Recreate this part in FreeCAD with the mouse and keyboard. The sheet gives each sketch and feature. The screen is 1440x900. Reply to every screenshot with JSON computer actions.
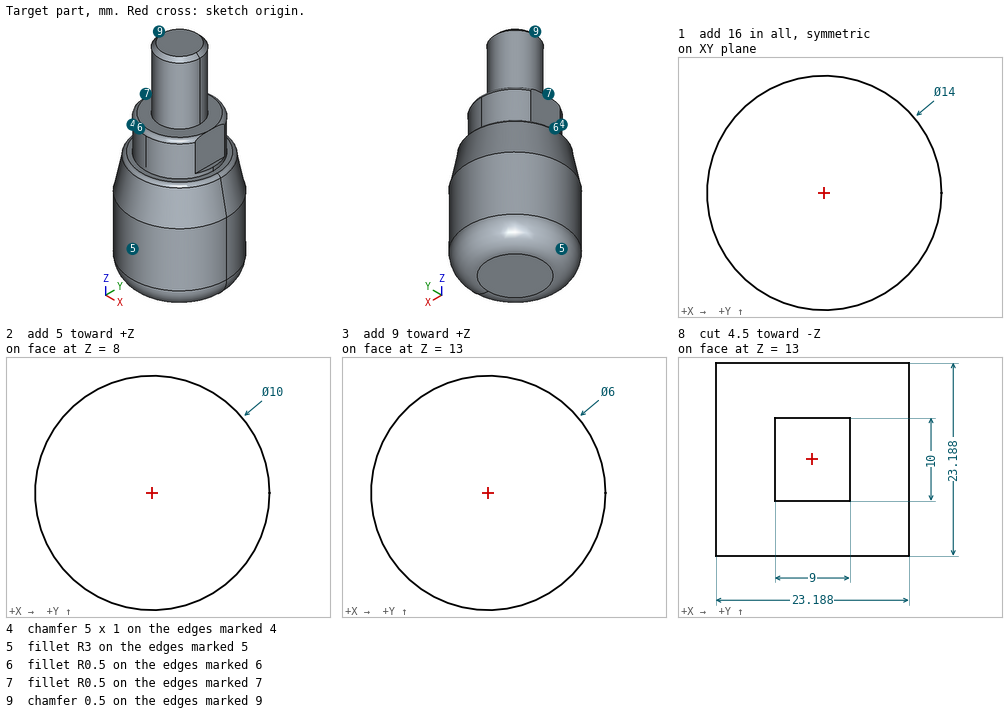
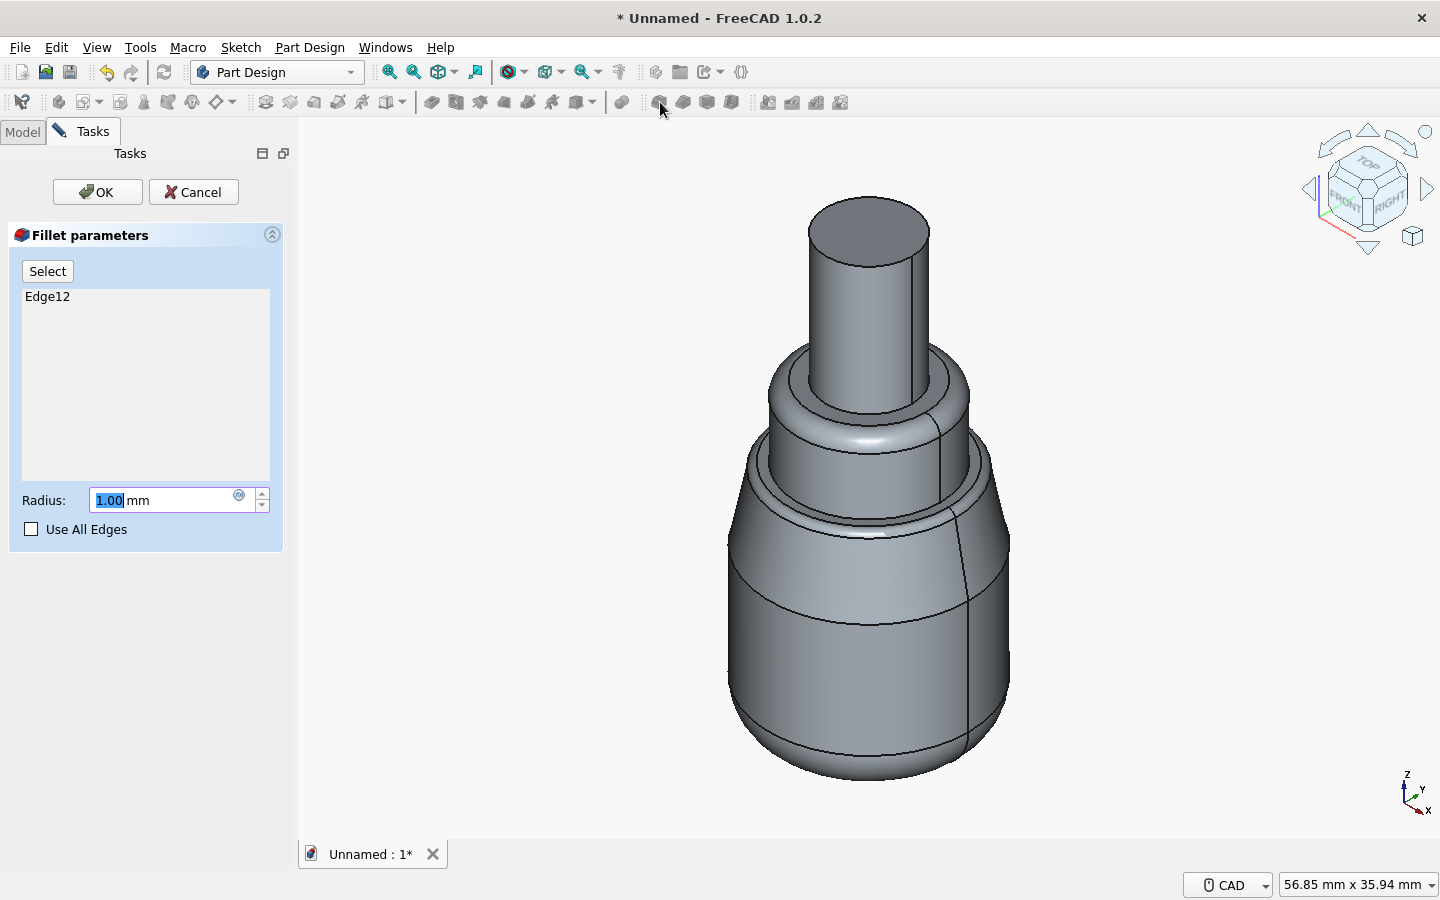
{"action": "type", "text": "0.5"}
{"action": "key", "text": "Tab"}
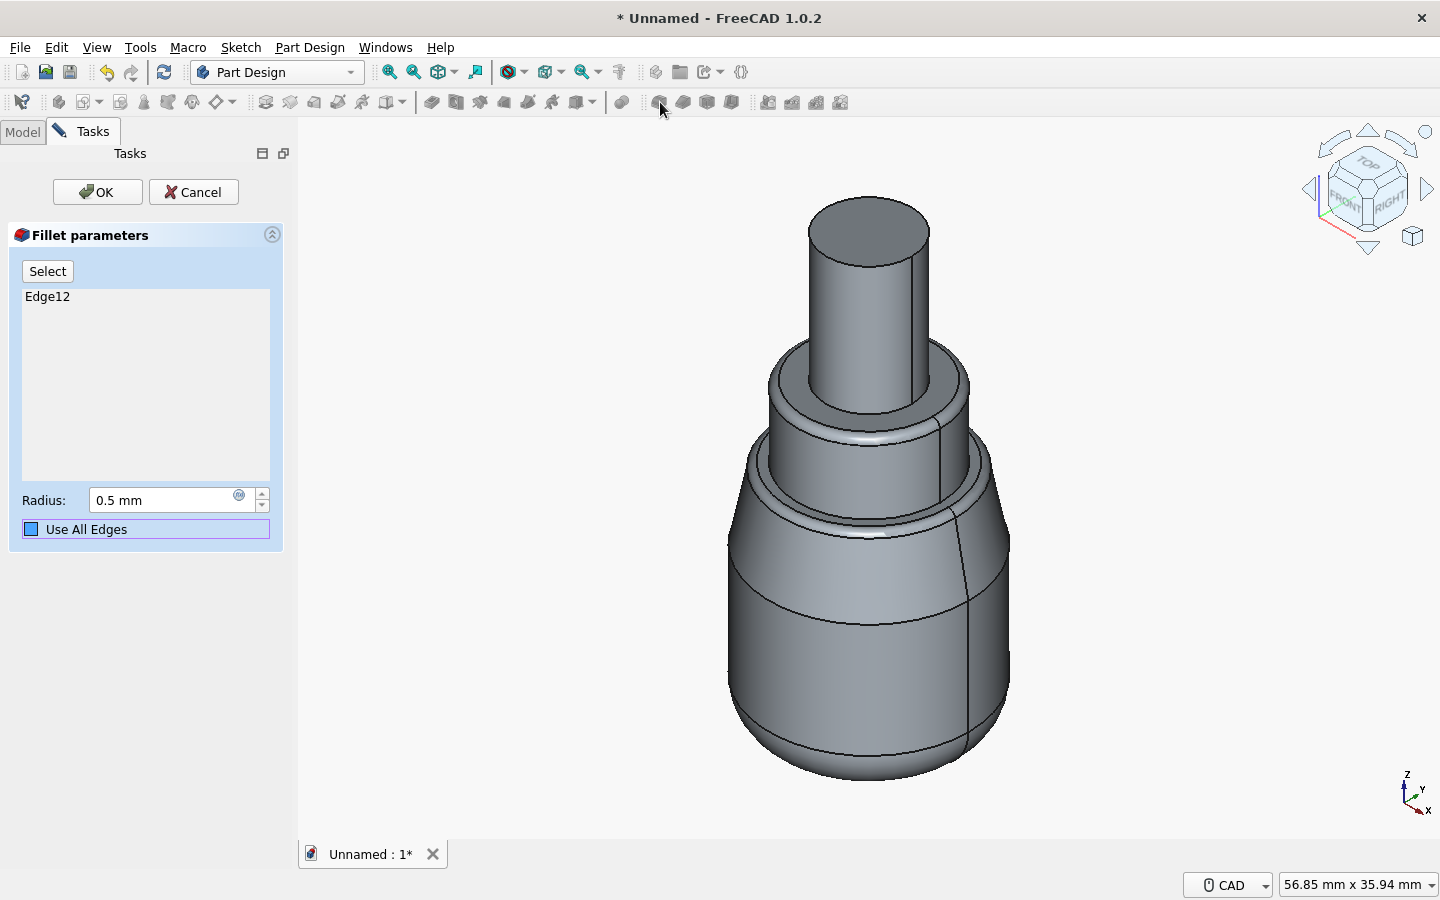
{"action": "left_click", "coordinate": [98, 192]}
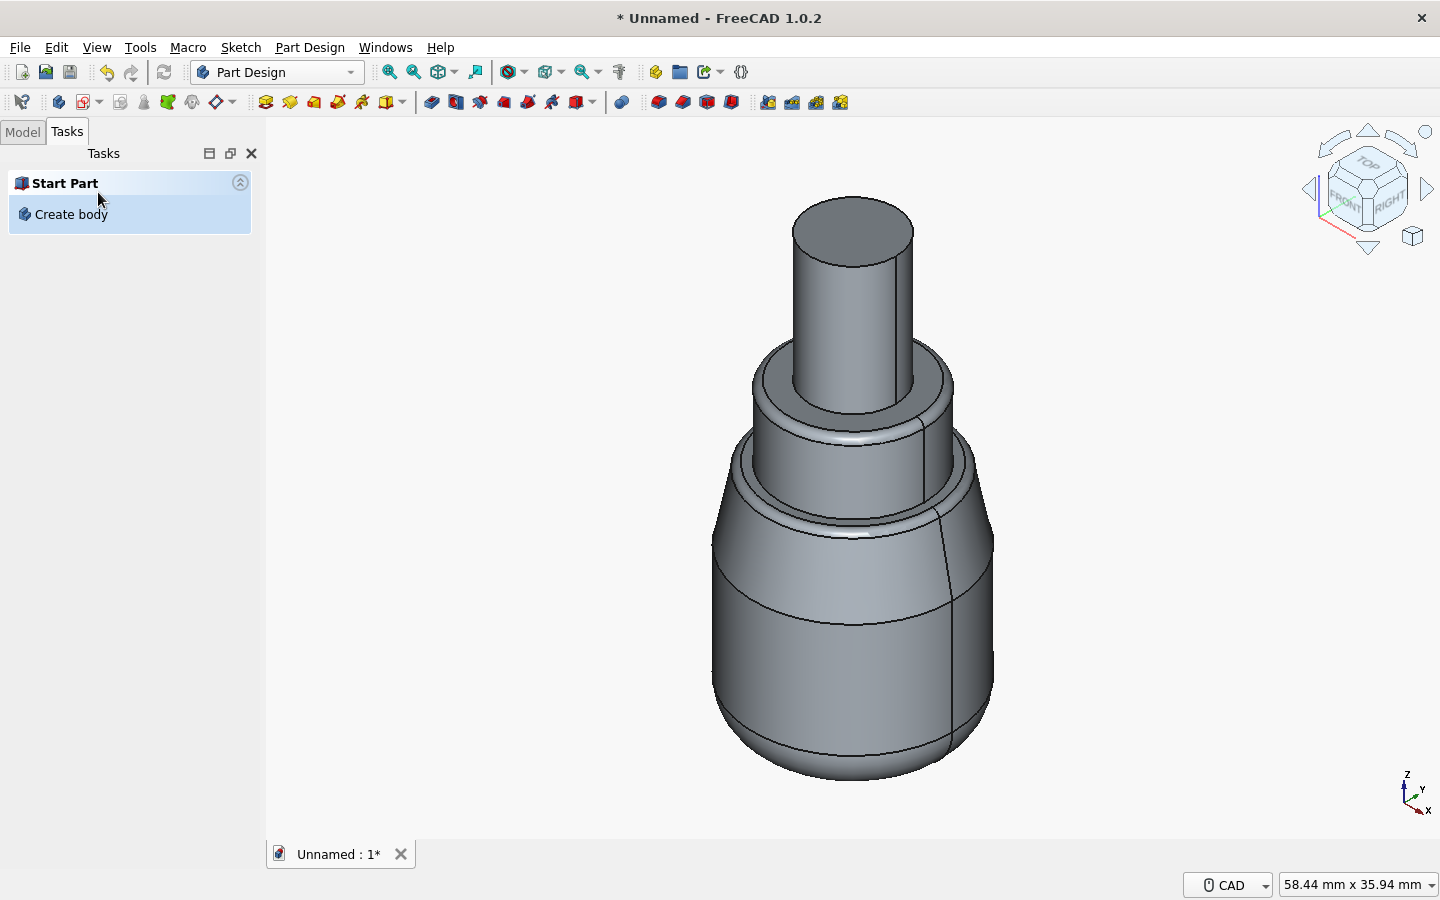
{"action": "key", "text": "v f"}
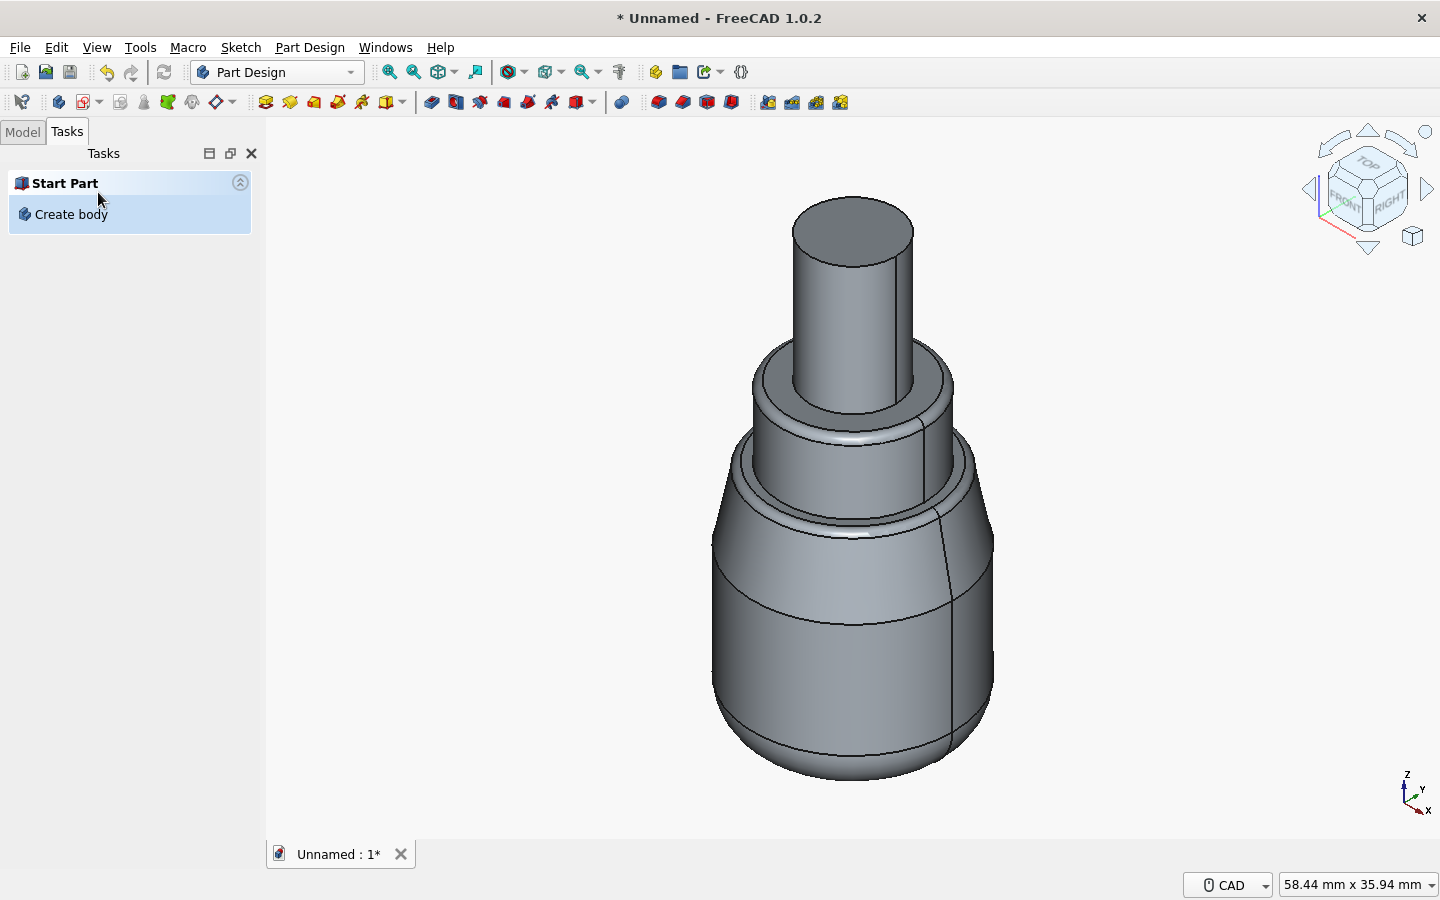
{"action": "left_click", "coordinate": [926, 379]}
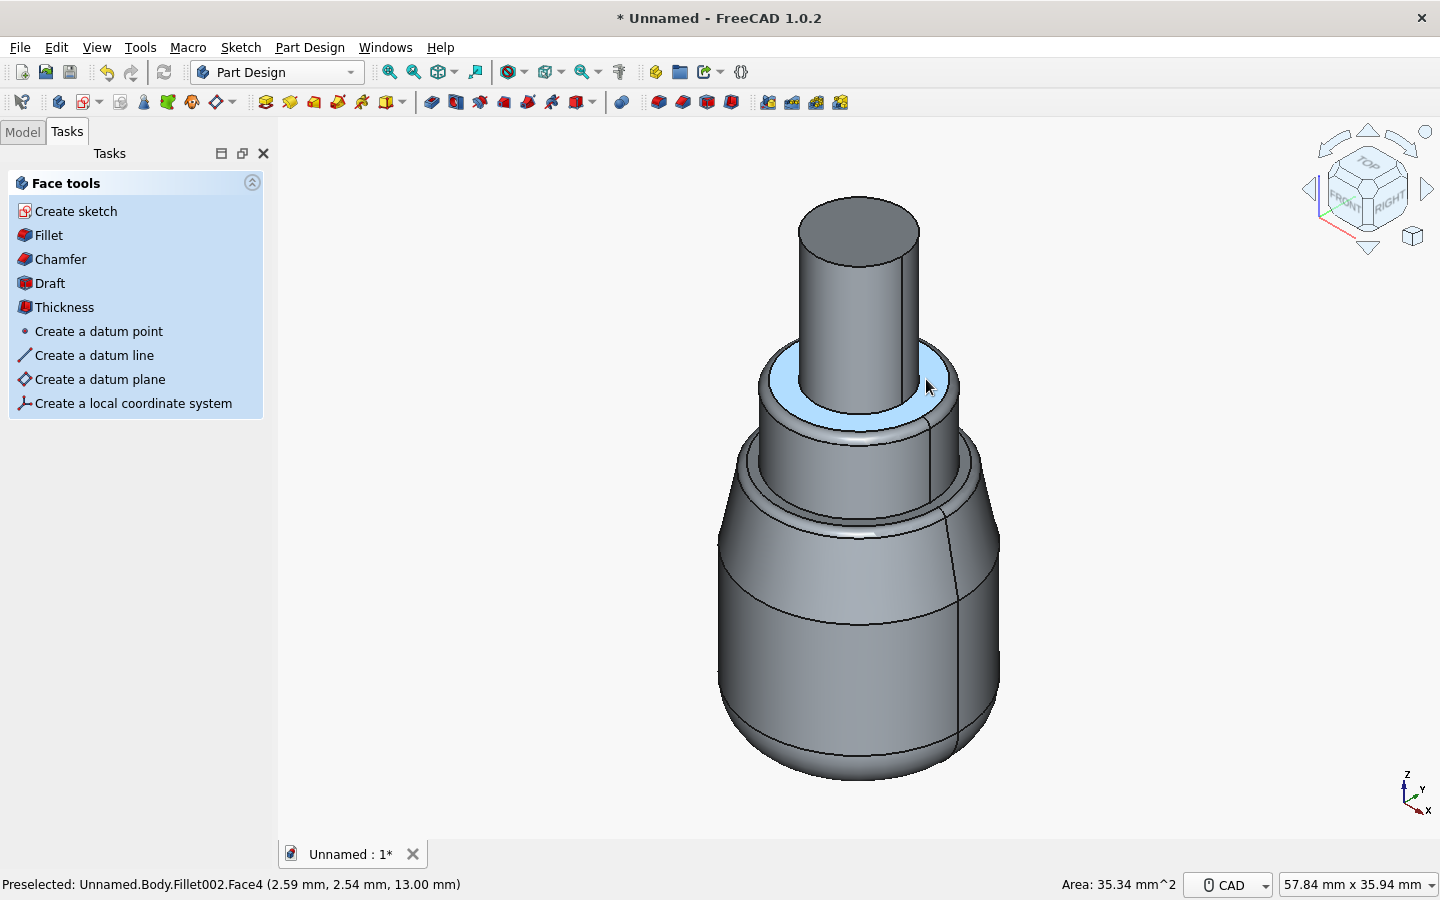
{"action": "left_click", "coordinate": [84, 102]}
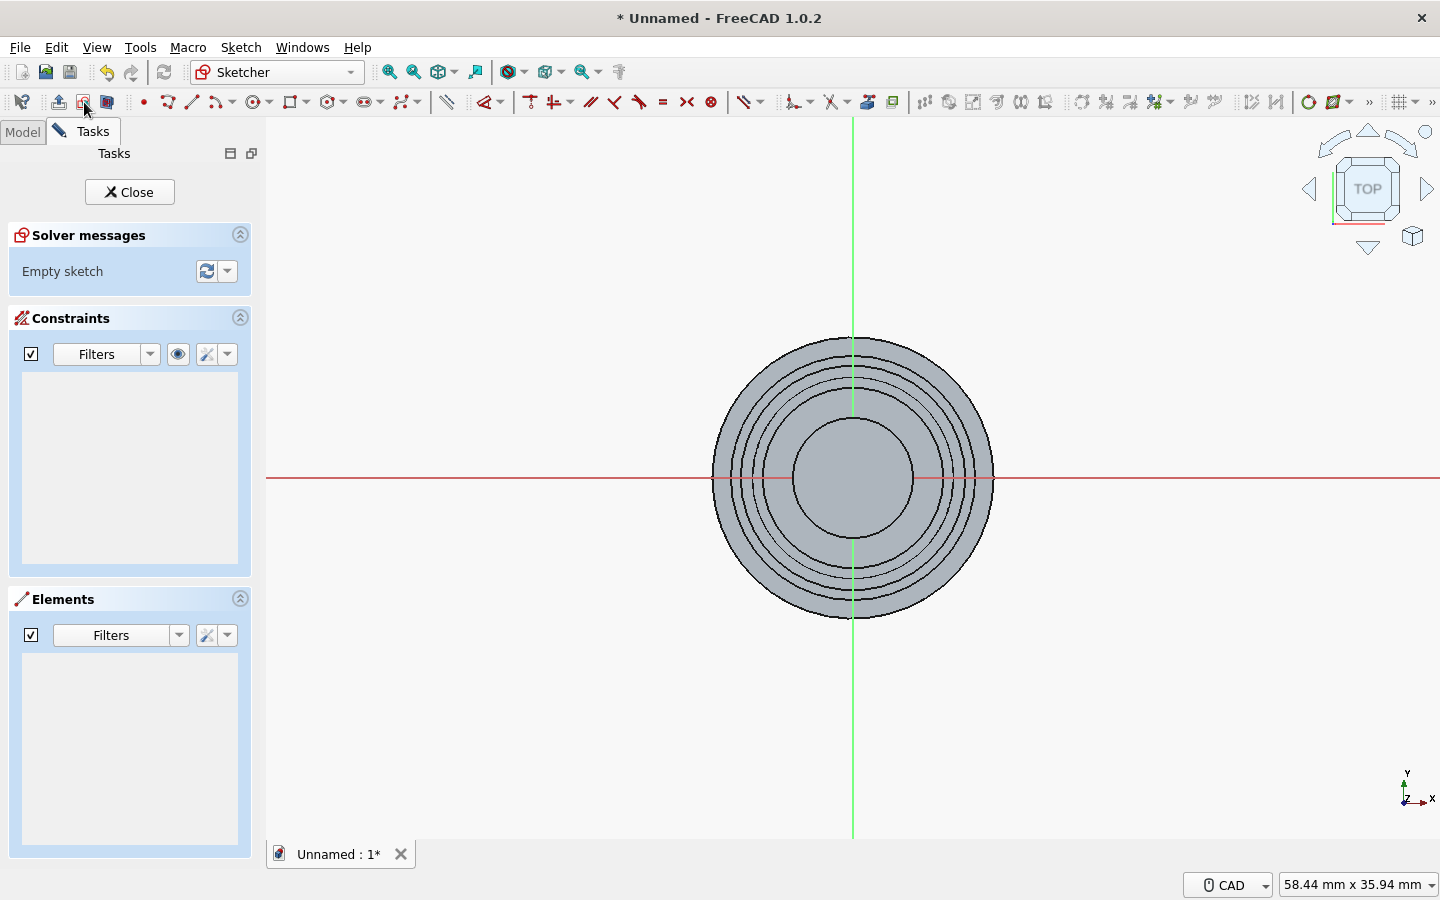
{"action": "key", "text": "g v"}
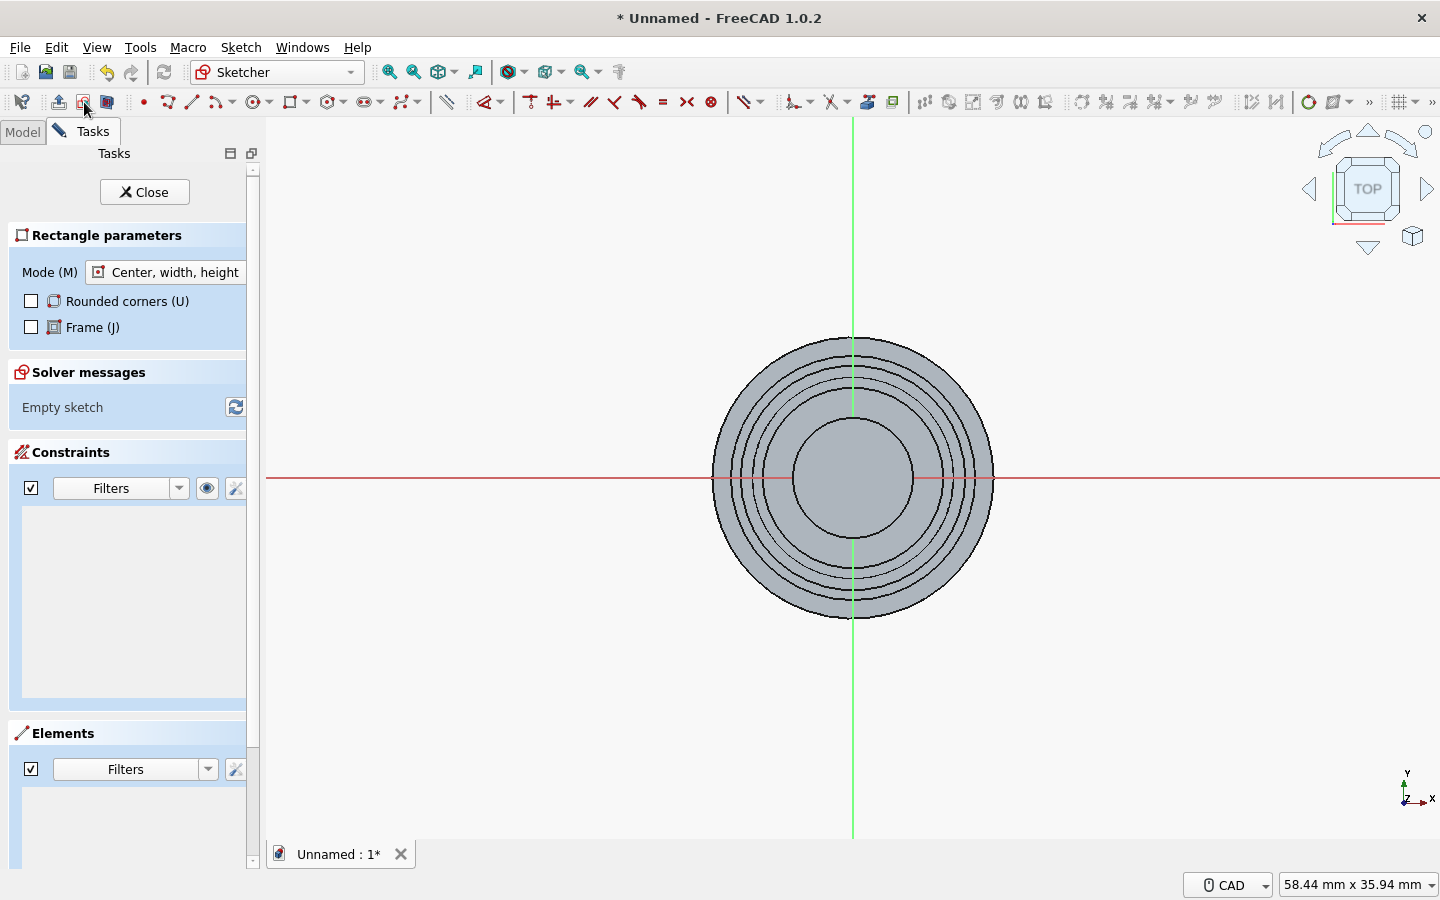
{"action": "left_click", "coordinate": [853, 478]}
{"action": "left_click", "coordinate": [1086, 245]}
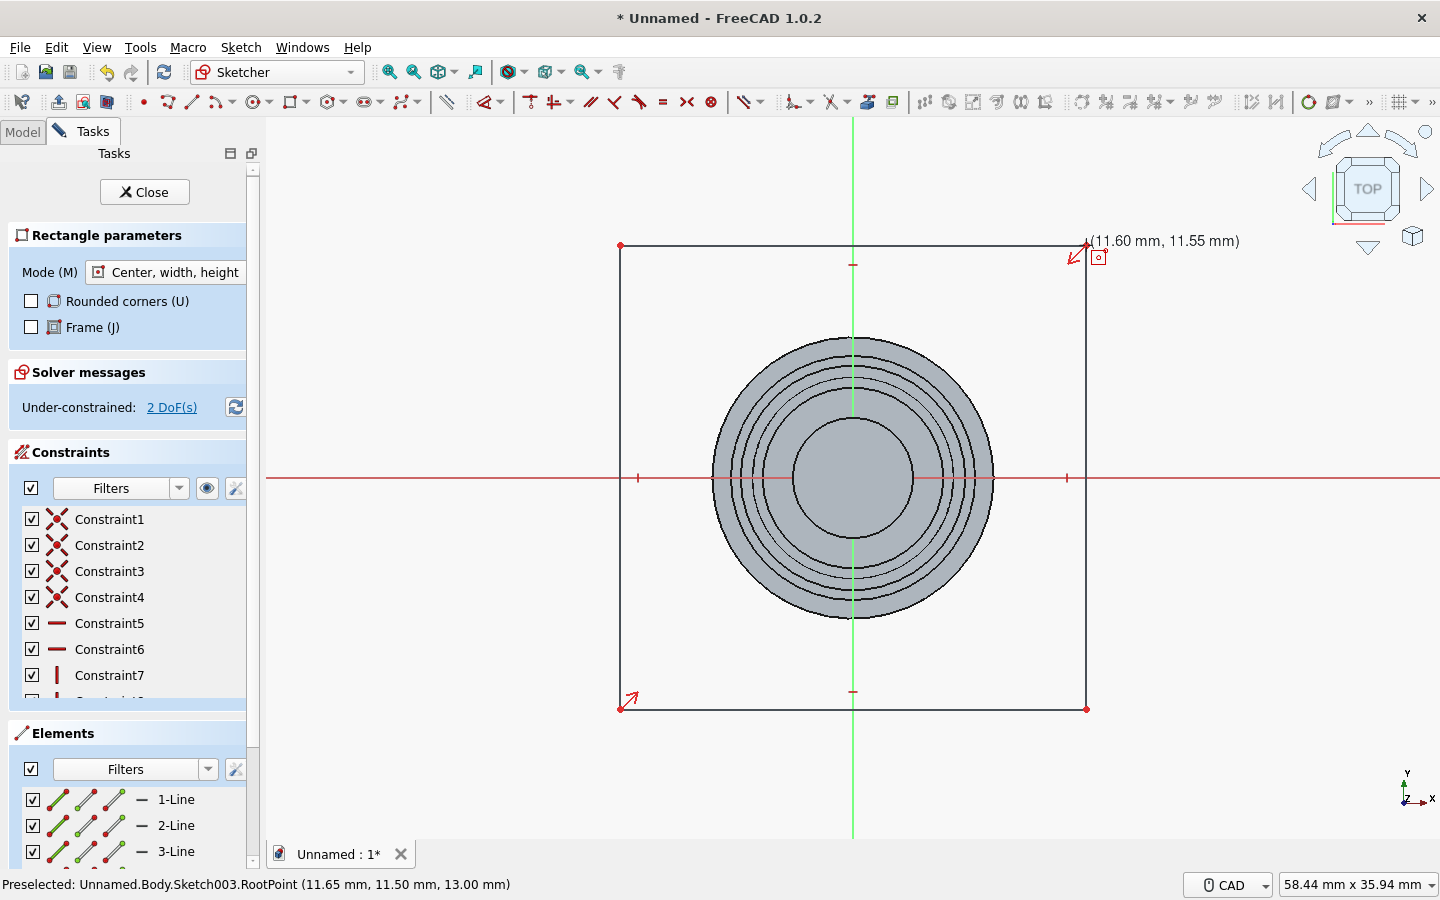
{"action": "left_click", "coordinate": [853, 478]}
{"action": "left_click", "coordinate": [943, 378]}
{"action": "key", "text": "Escape"}